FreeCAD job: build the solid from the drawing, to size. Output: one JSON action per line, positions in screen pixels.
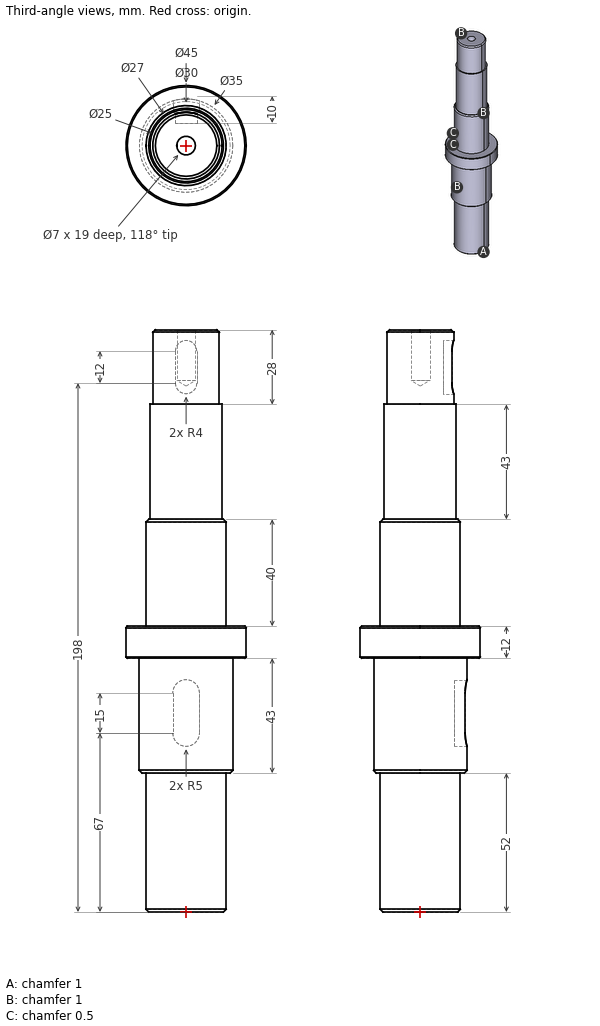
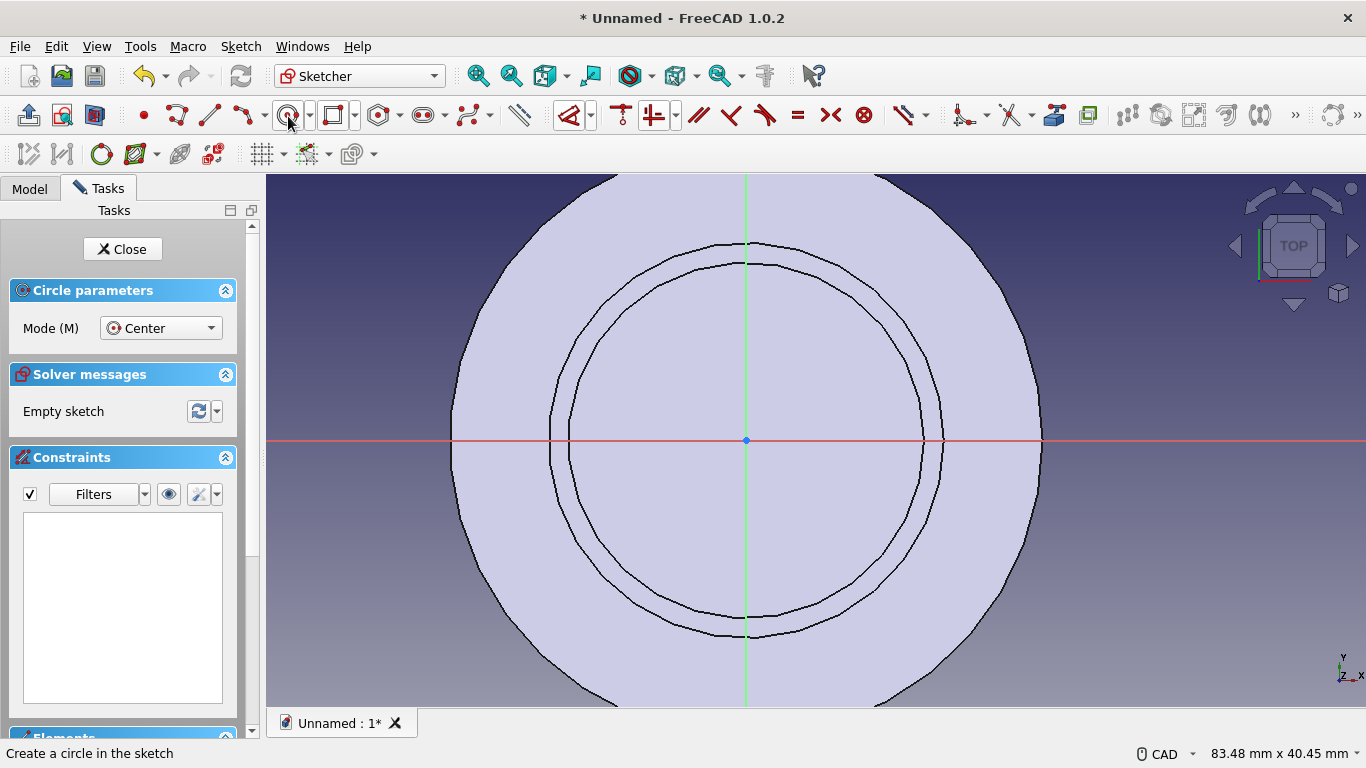
{"action": "left_click", "coordinate": [746, 440]}
{"action": "mouse_move", "coordinate": [863, 324]}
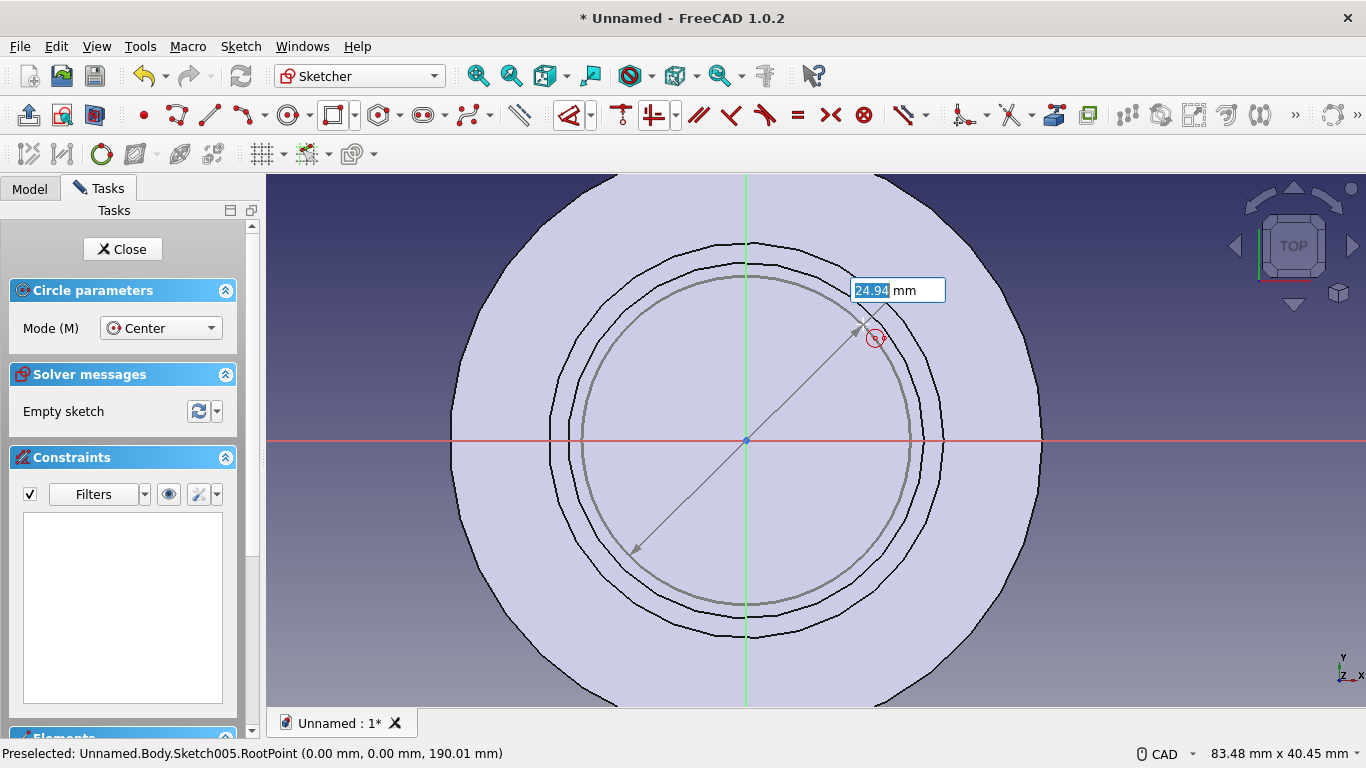
{"action": "type", "text": "25"}
{"action": "key", "text": "Return"}
{"action": "key", "text": "Escape"}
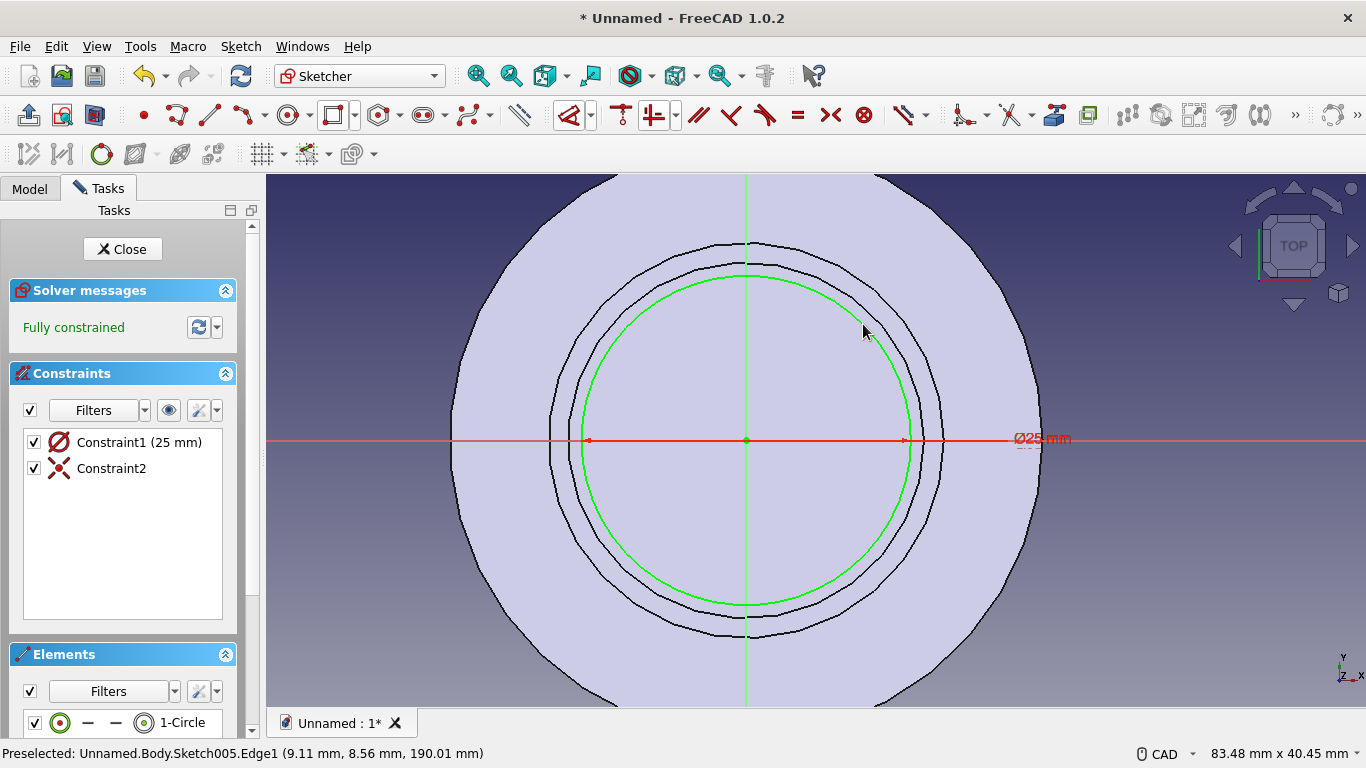
{"action": "left_click", "coordinate": [123, 249]}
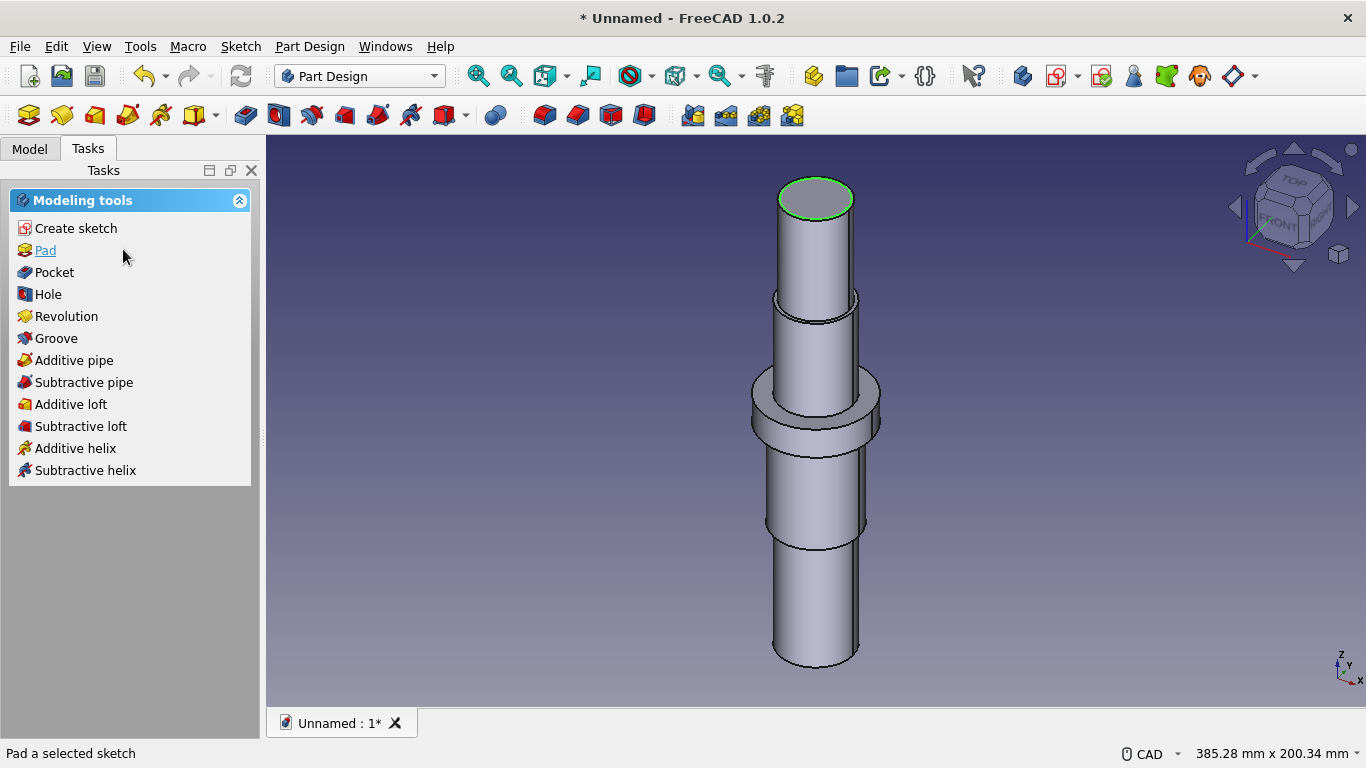
{"action": "left_click", "coordinate": [29, 116]}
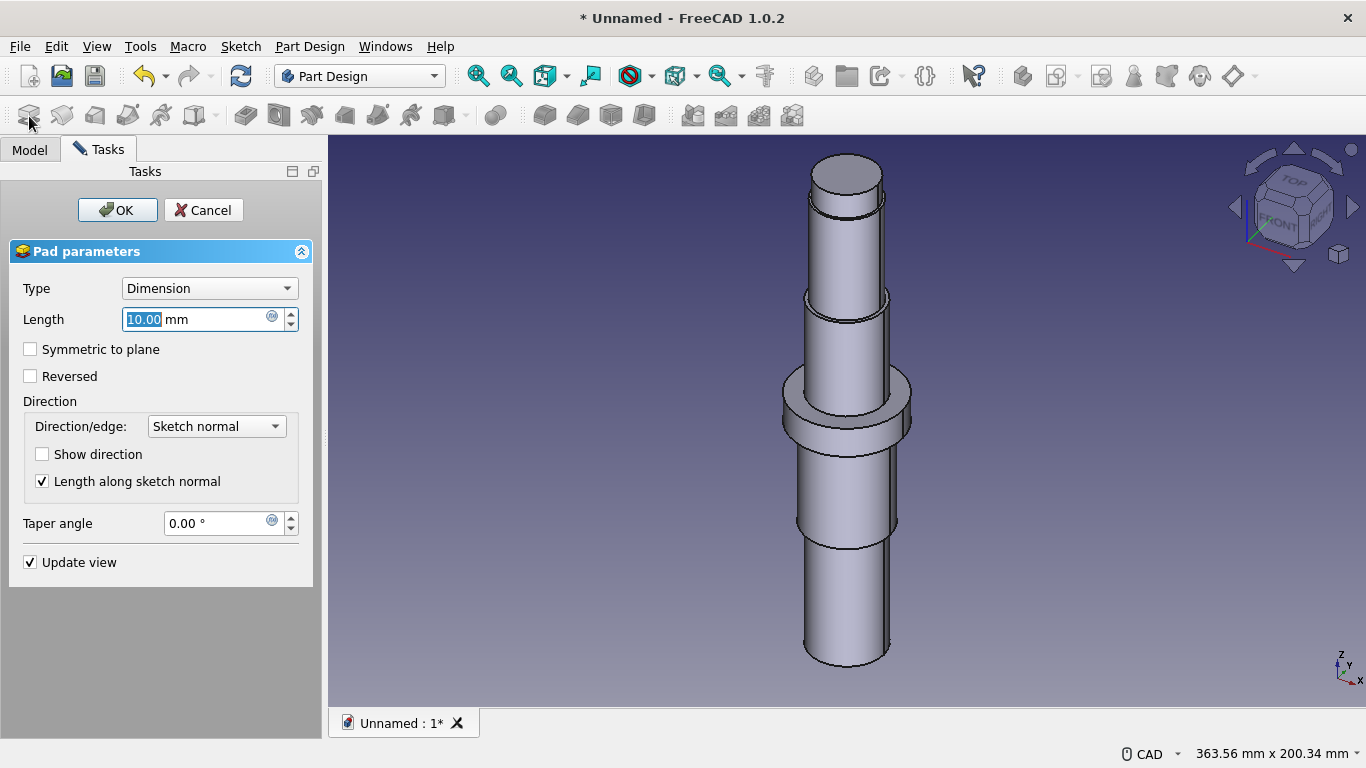
{"action": "type", "text": "28"}
{"action": "key", "text": "Tab"}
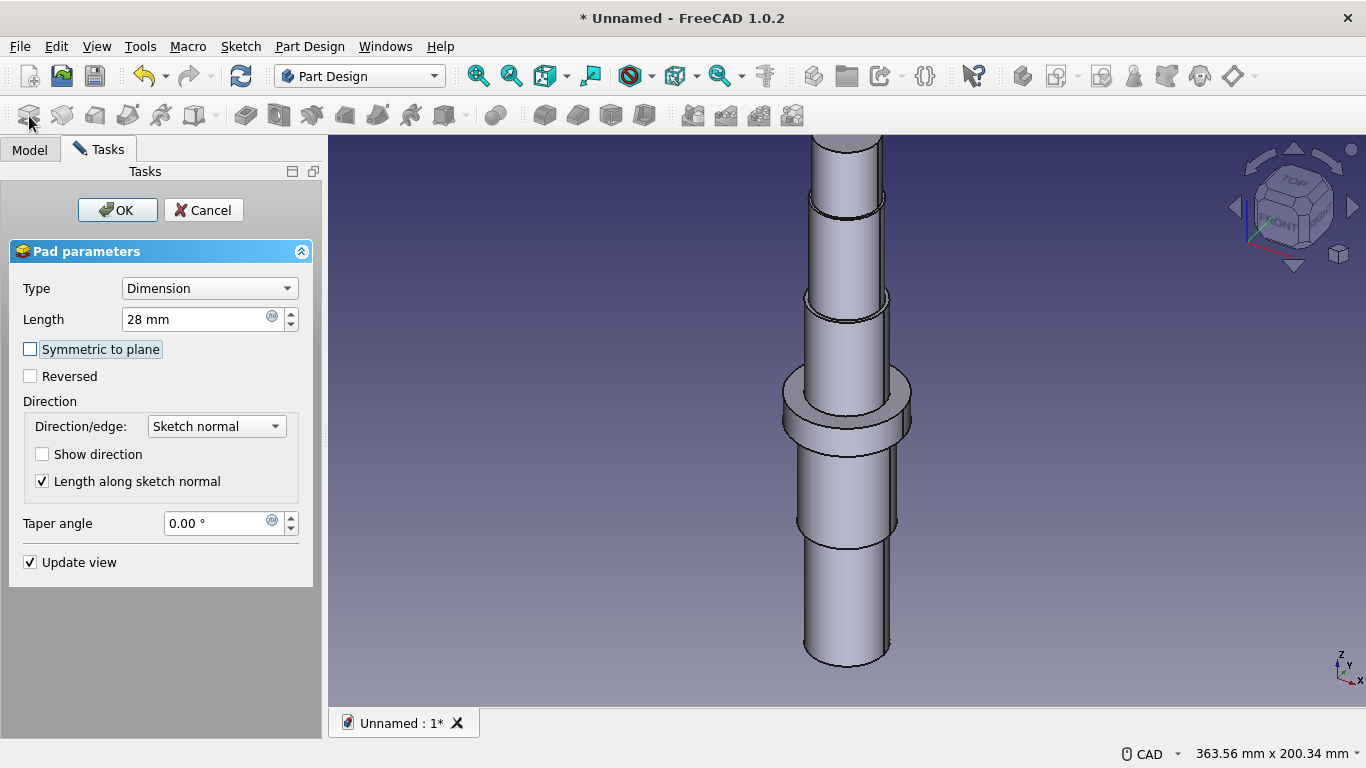
{"action": "left_click", "coordinate": [118, 210]}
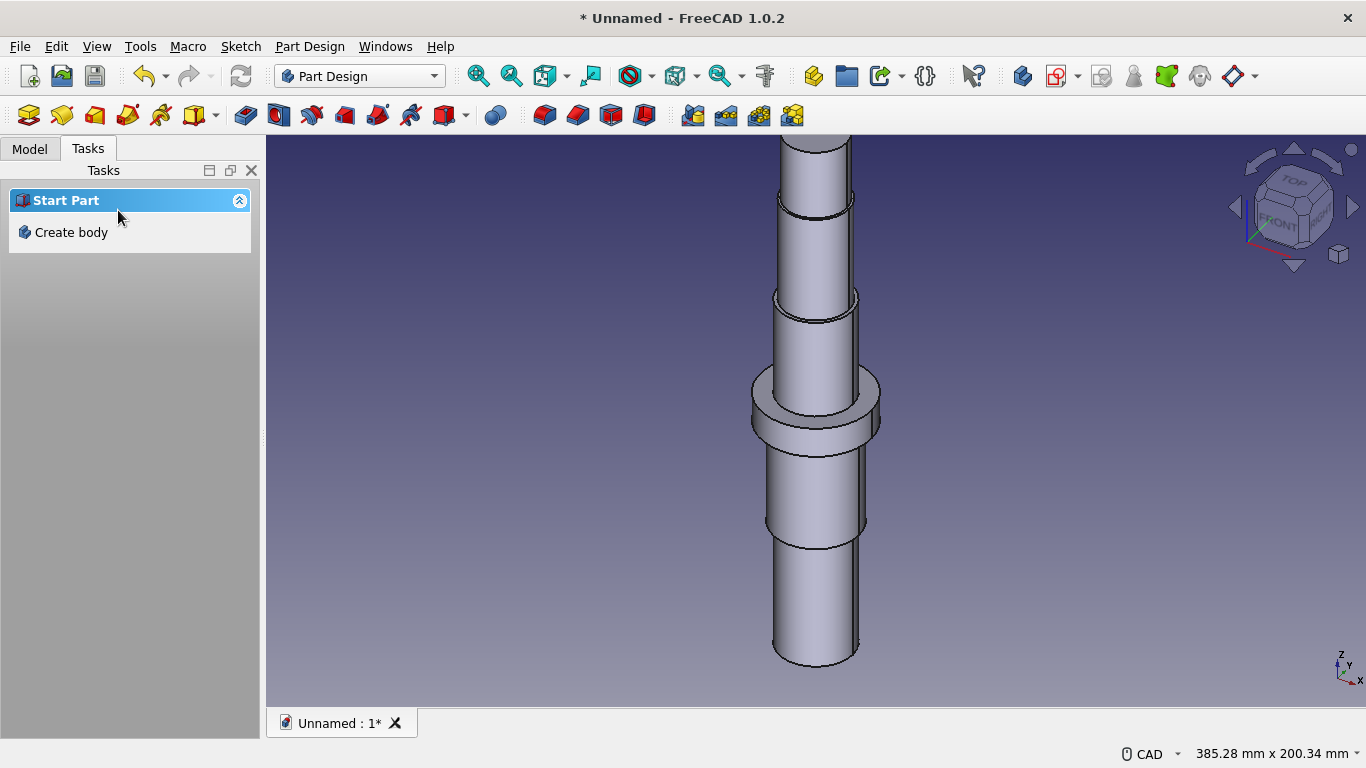
{"action": "key", "text": "v f"}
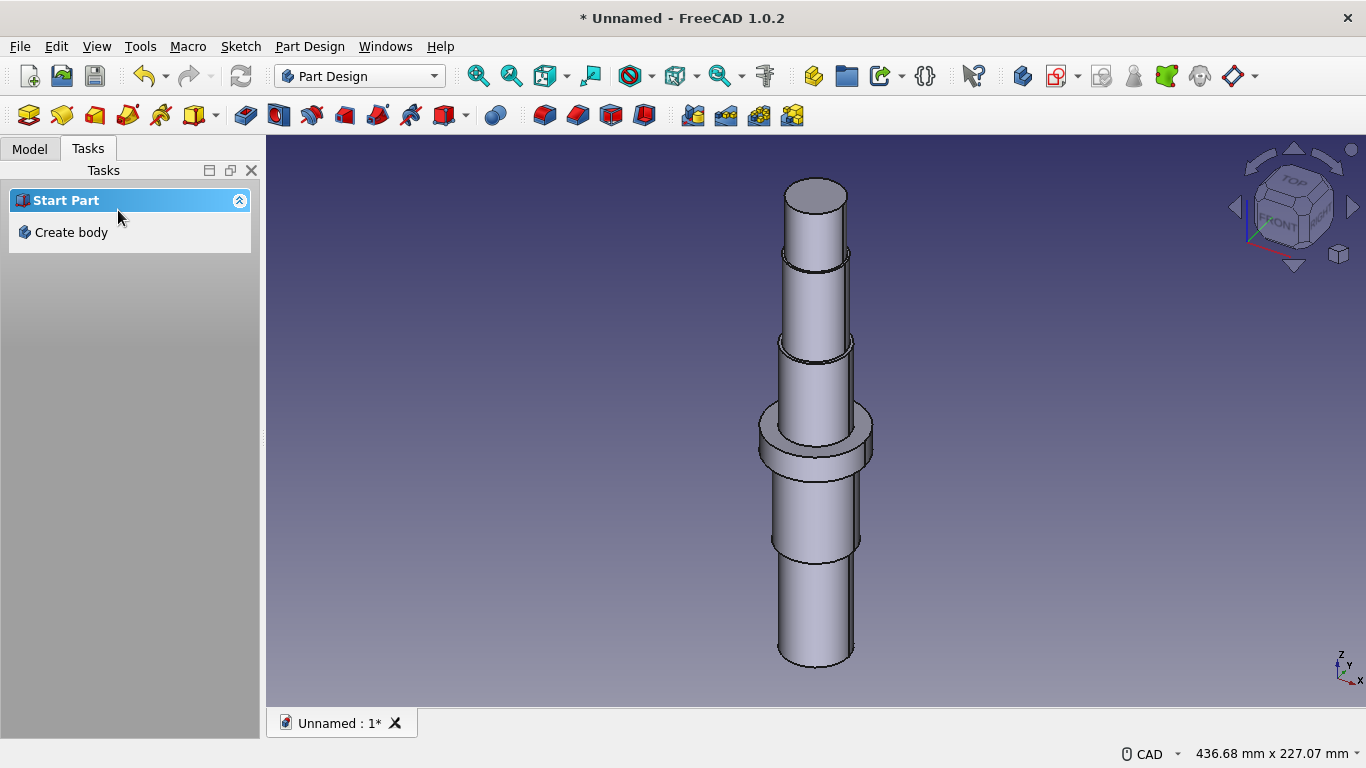
{"action": "key", "text": "0"}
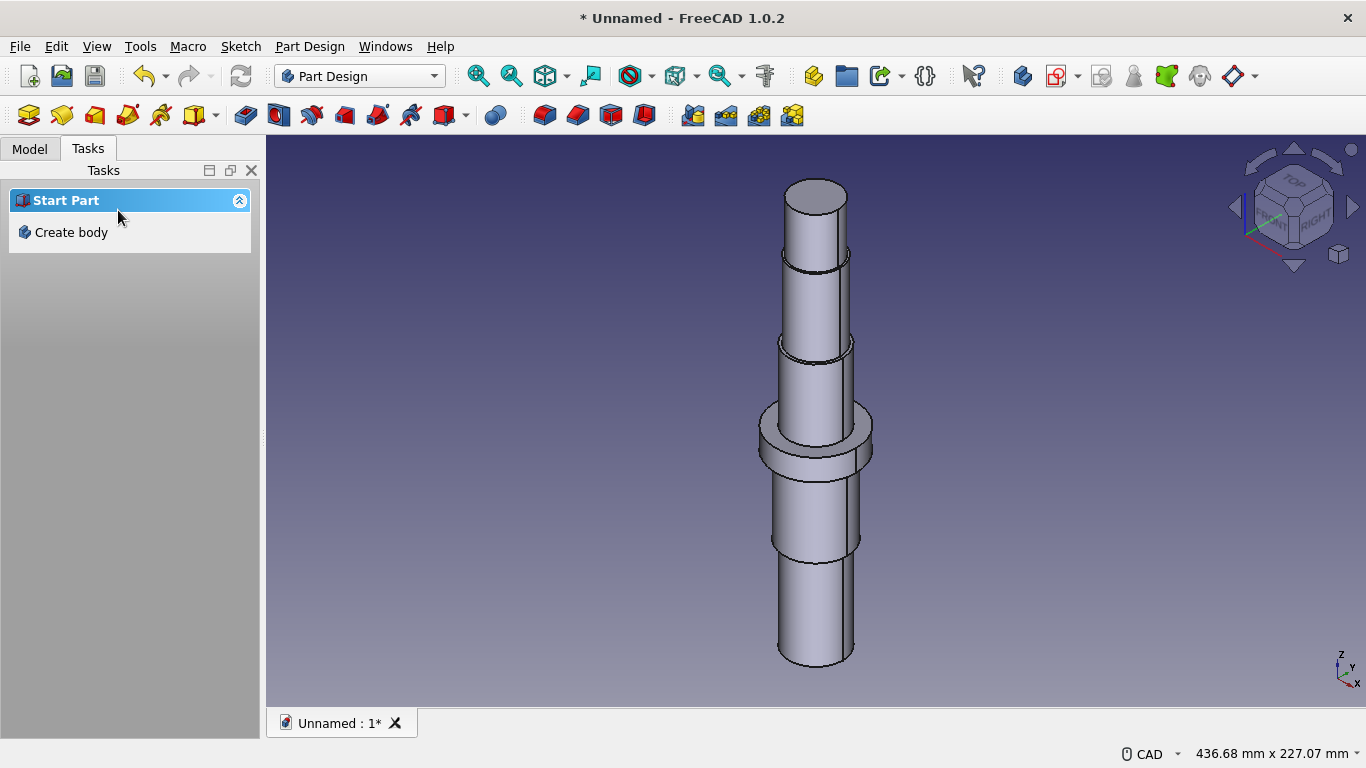
{"action": "key", "text": "2"}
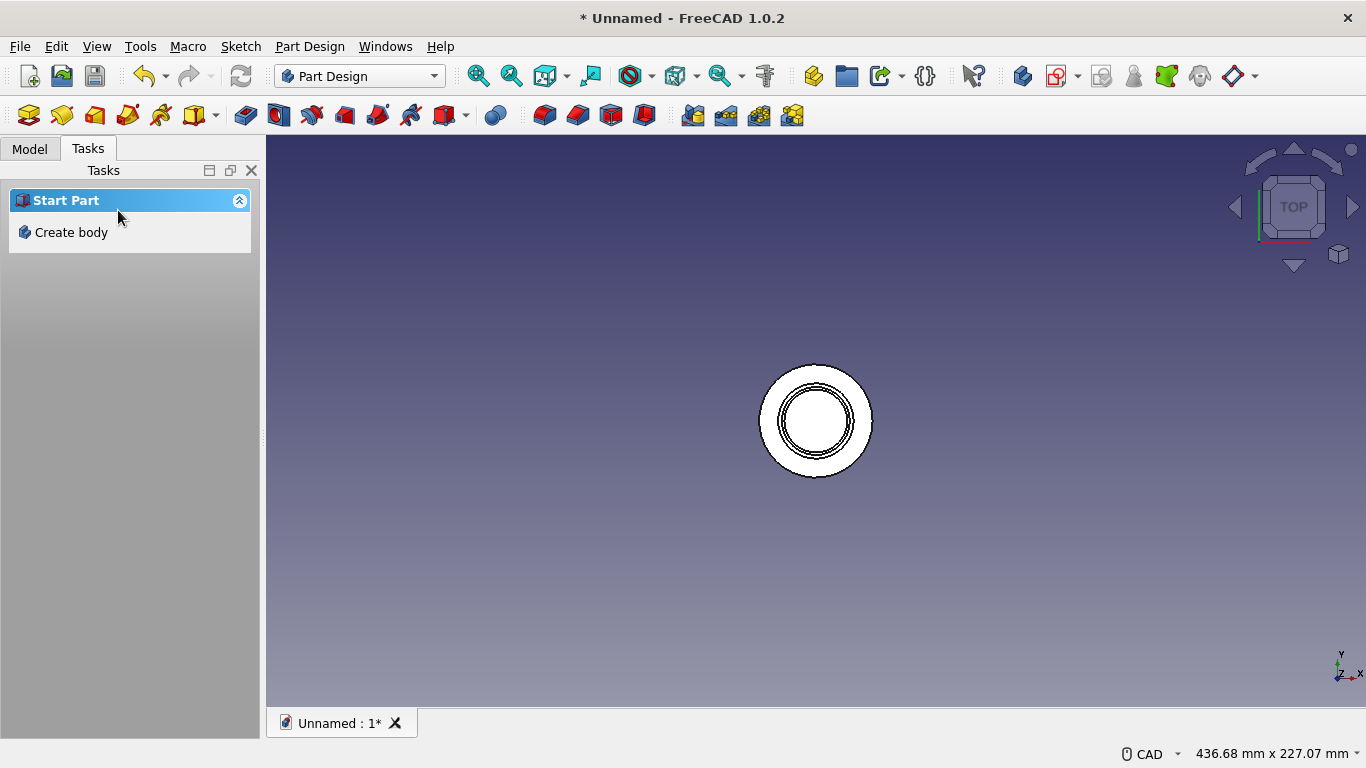
{"action": "key", "text": "v f"}